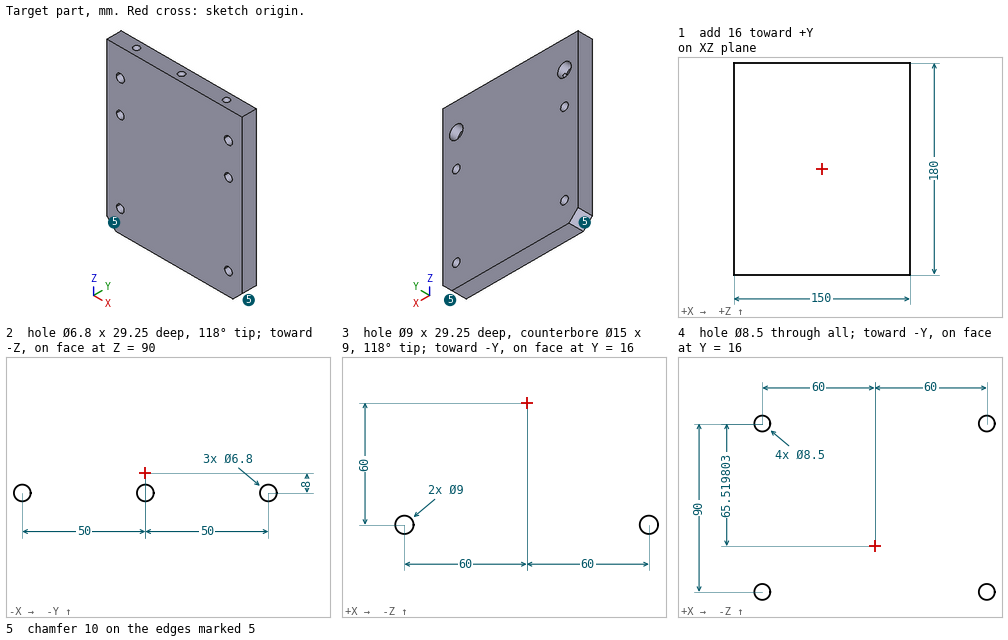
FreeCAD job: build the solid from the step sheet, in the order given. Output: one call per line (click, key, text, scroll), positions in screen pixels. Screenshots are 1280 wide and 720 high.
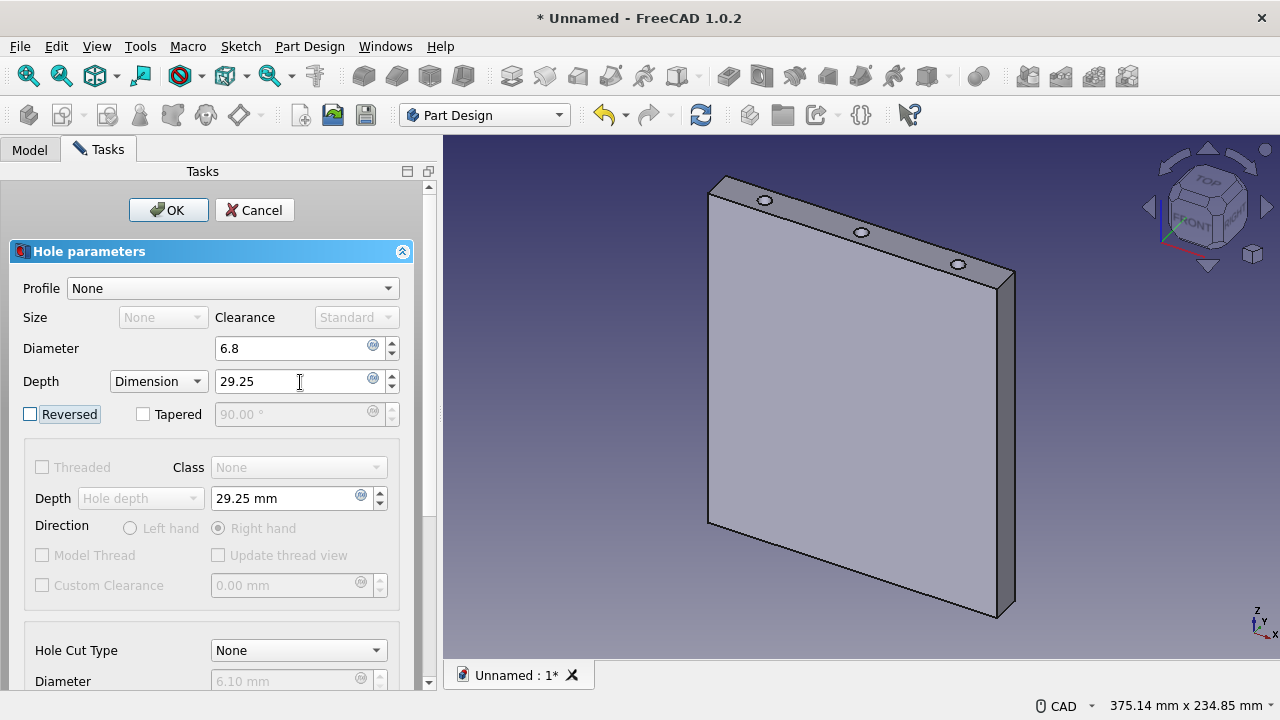
click(169, 210)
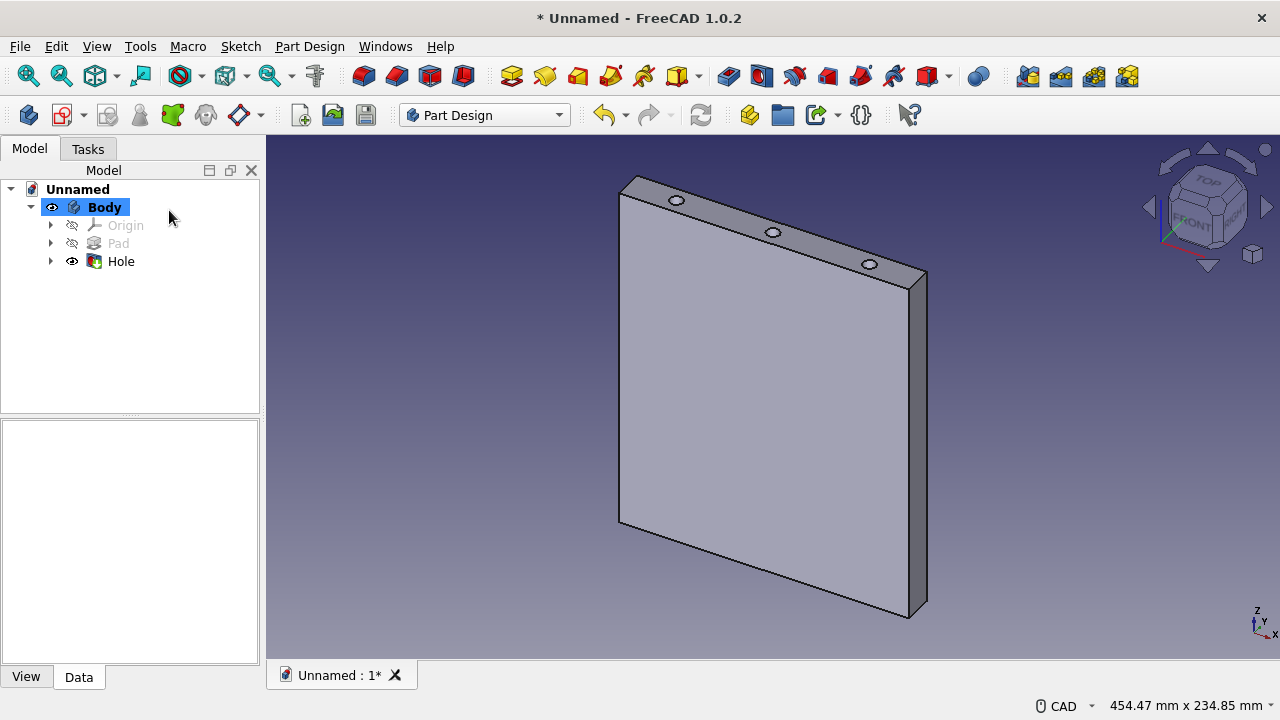
key(4)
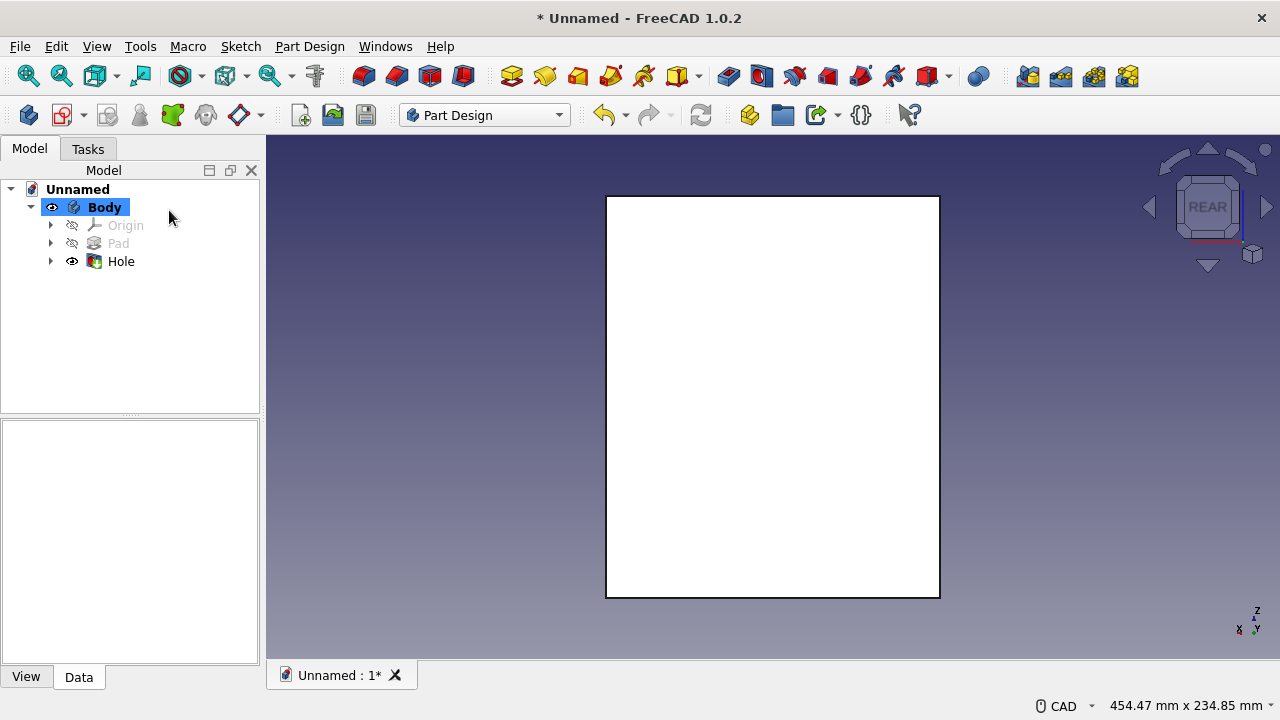
click(773, 396)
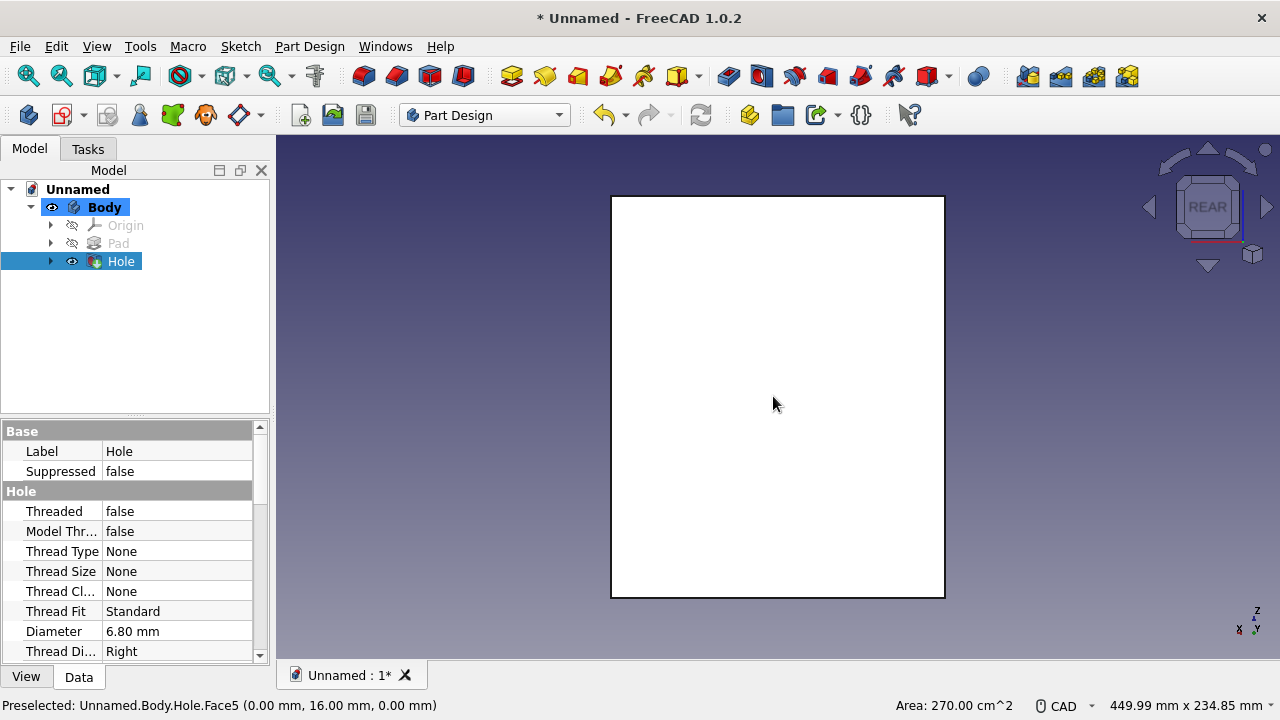
click(62, 116)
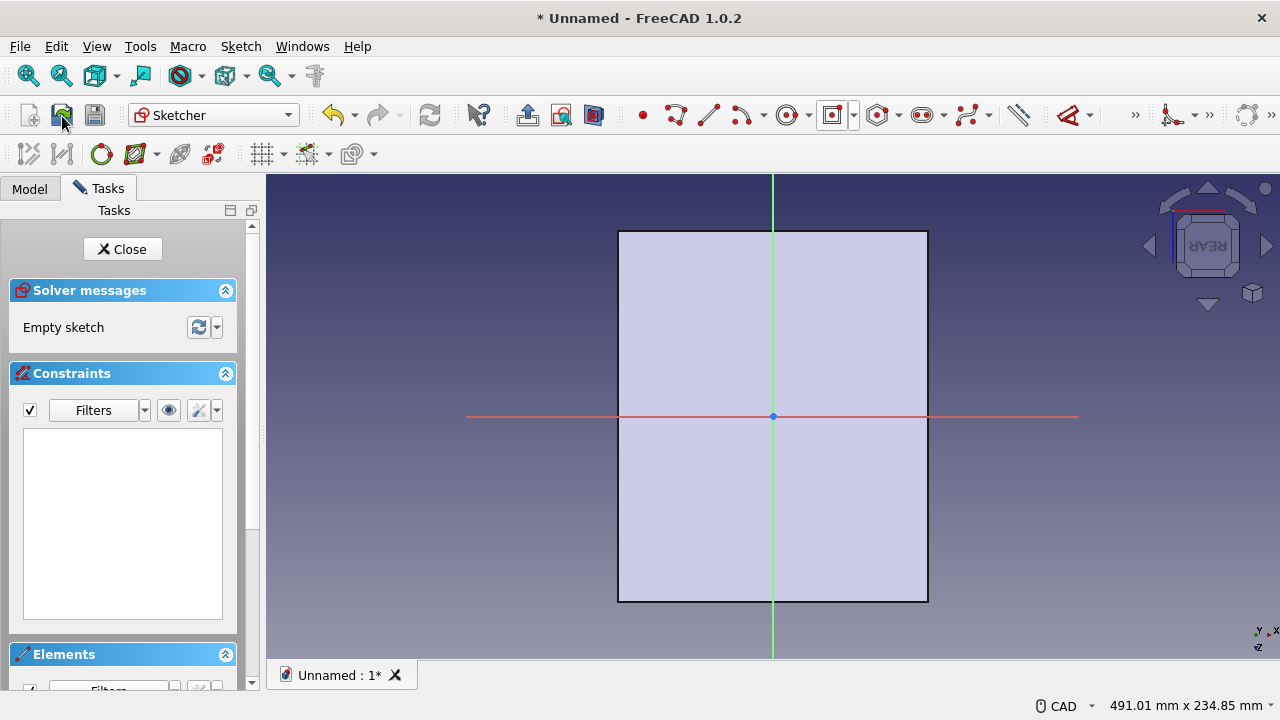
scroll(829, 537, up, 4)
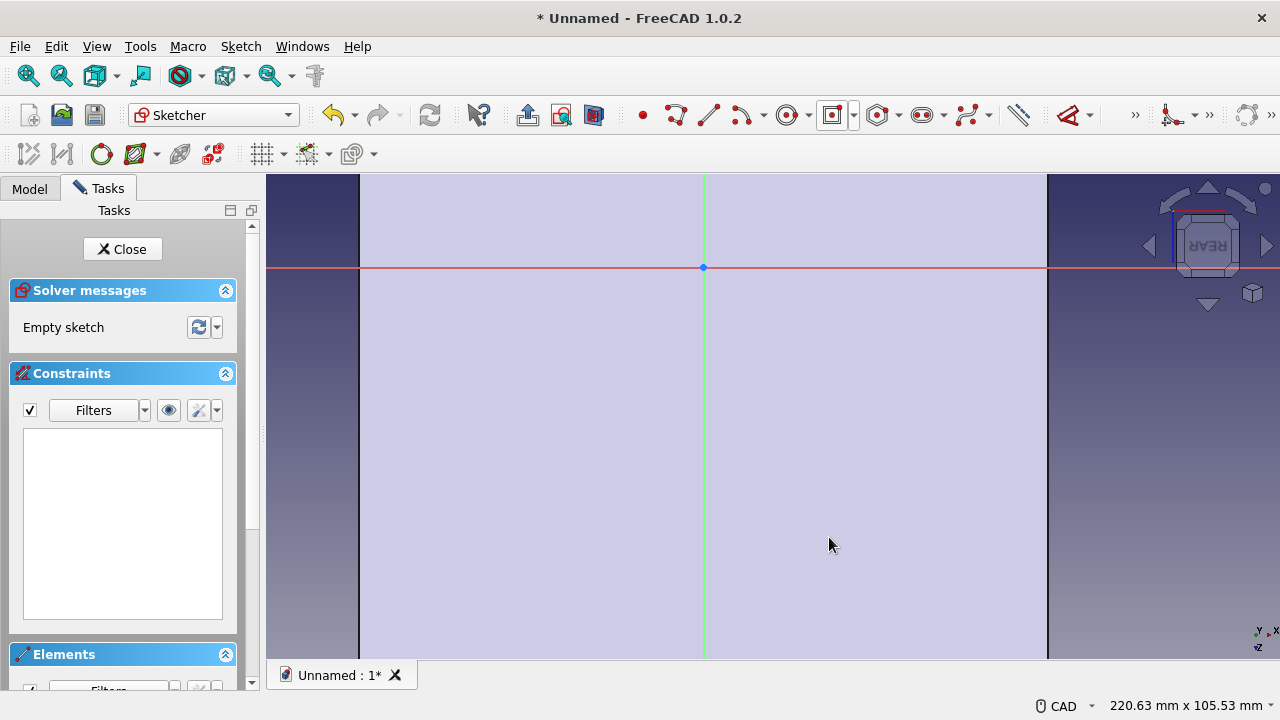
click(786, 116)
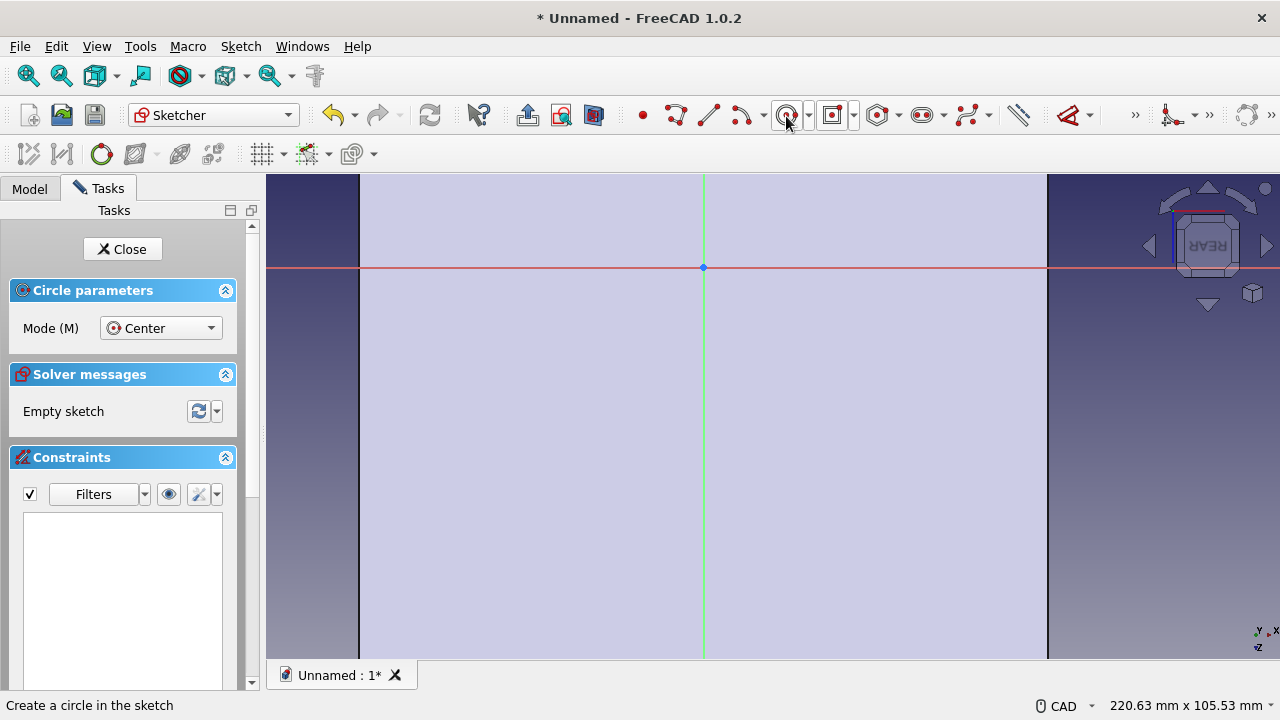
click(428, 544)
move(443, 529)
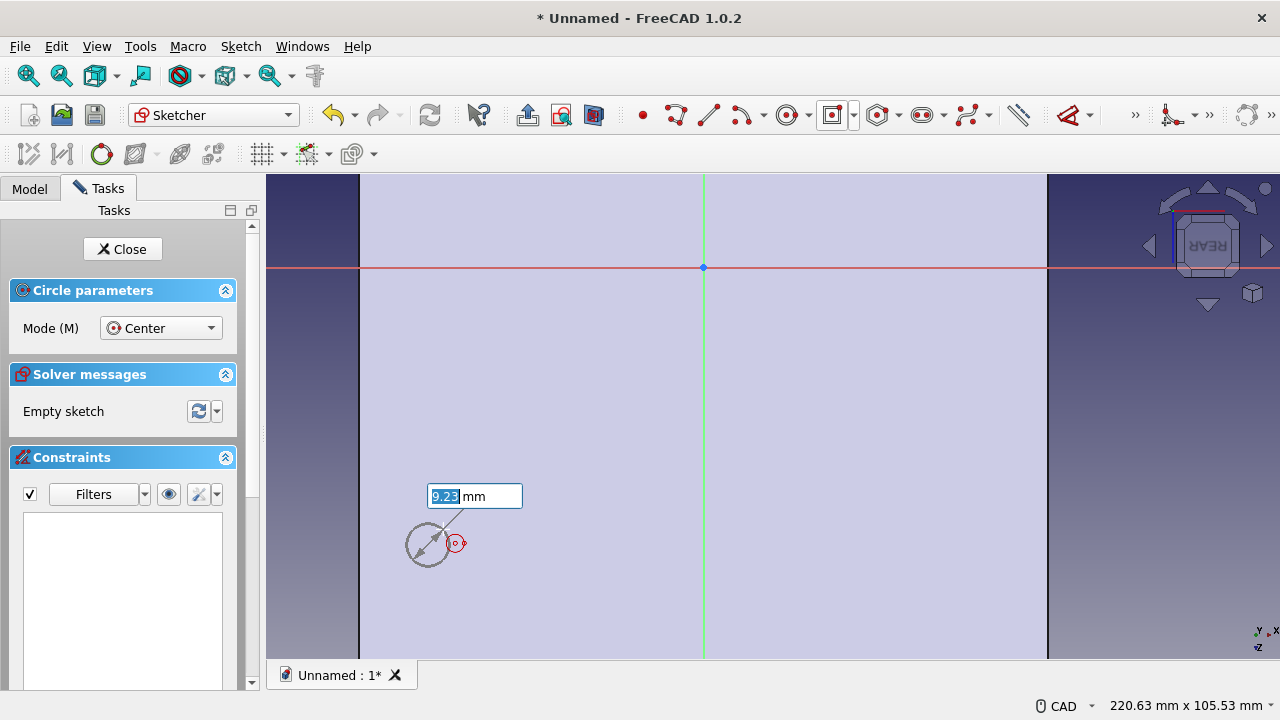
text(9)
key(Return)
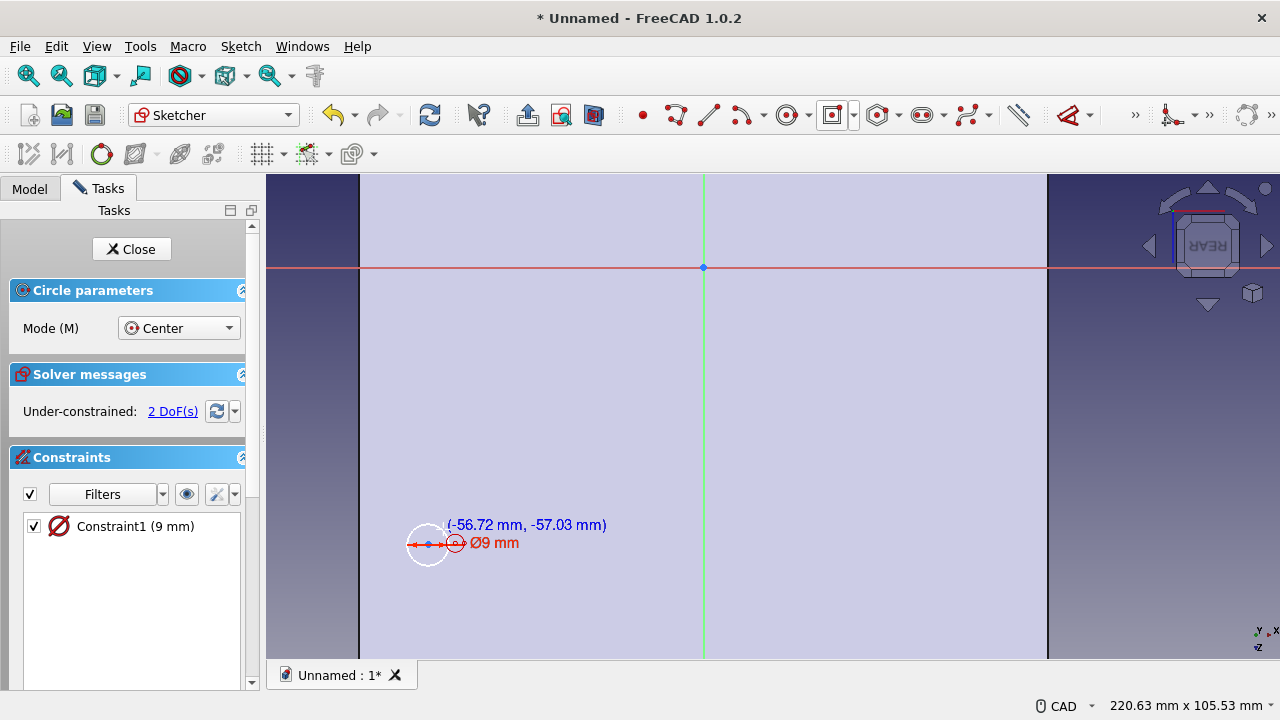
click(979, 544)
move(994, 529)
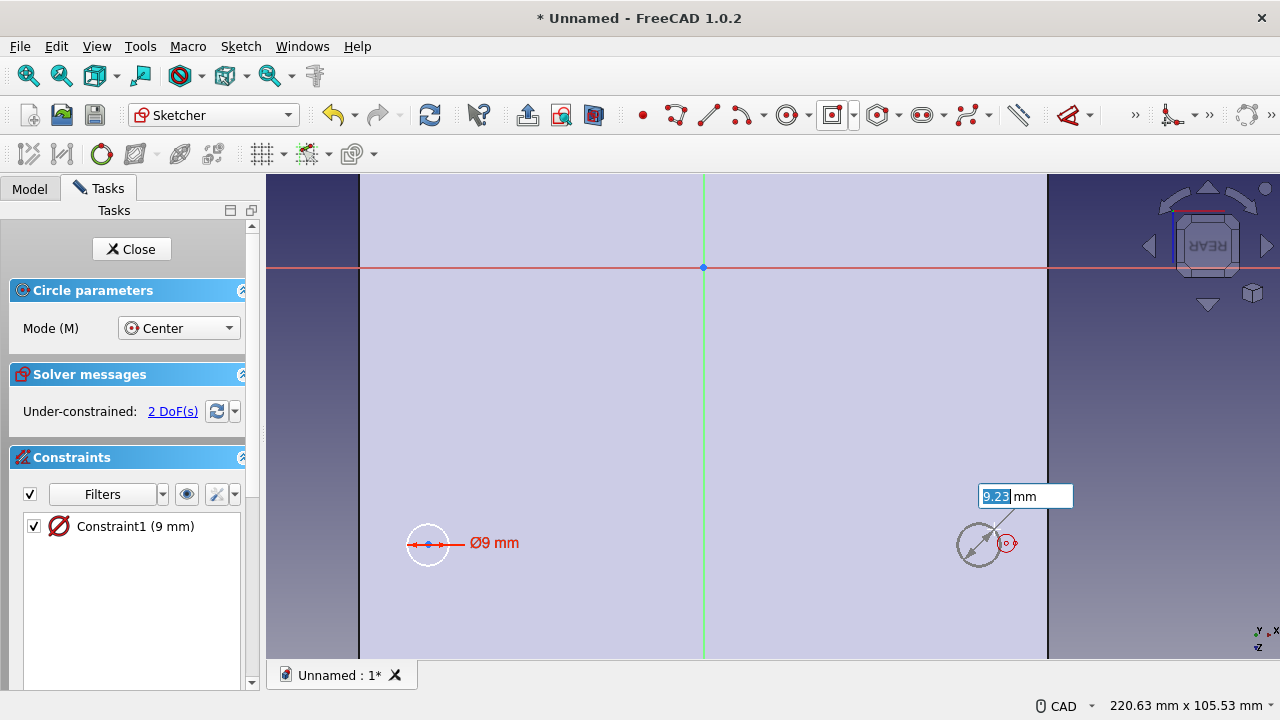
text(9)
key(Return)
key(Escape)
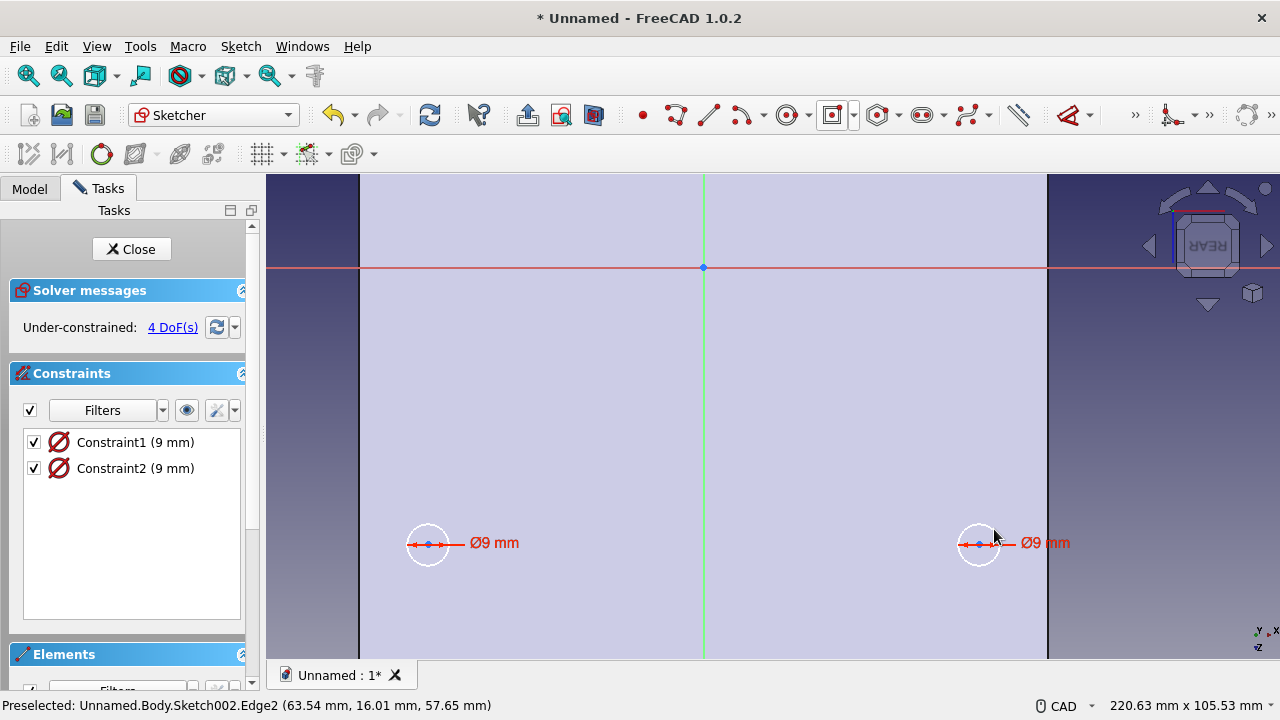
click(428, 545)